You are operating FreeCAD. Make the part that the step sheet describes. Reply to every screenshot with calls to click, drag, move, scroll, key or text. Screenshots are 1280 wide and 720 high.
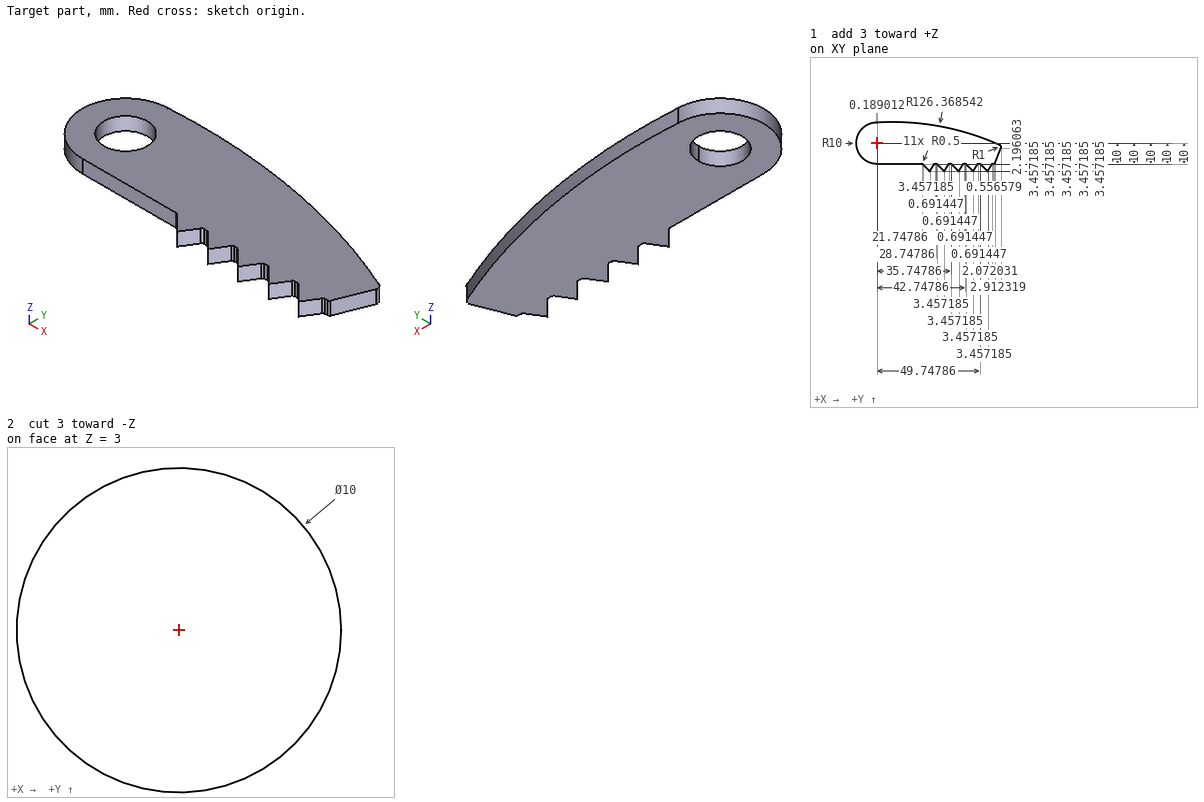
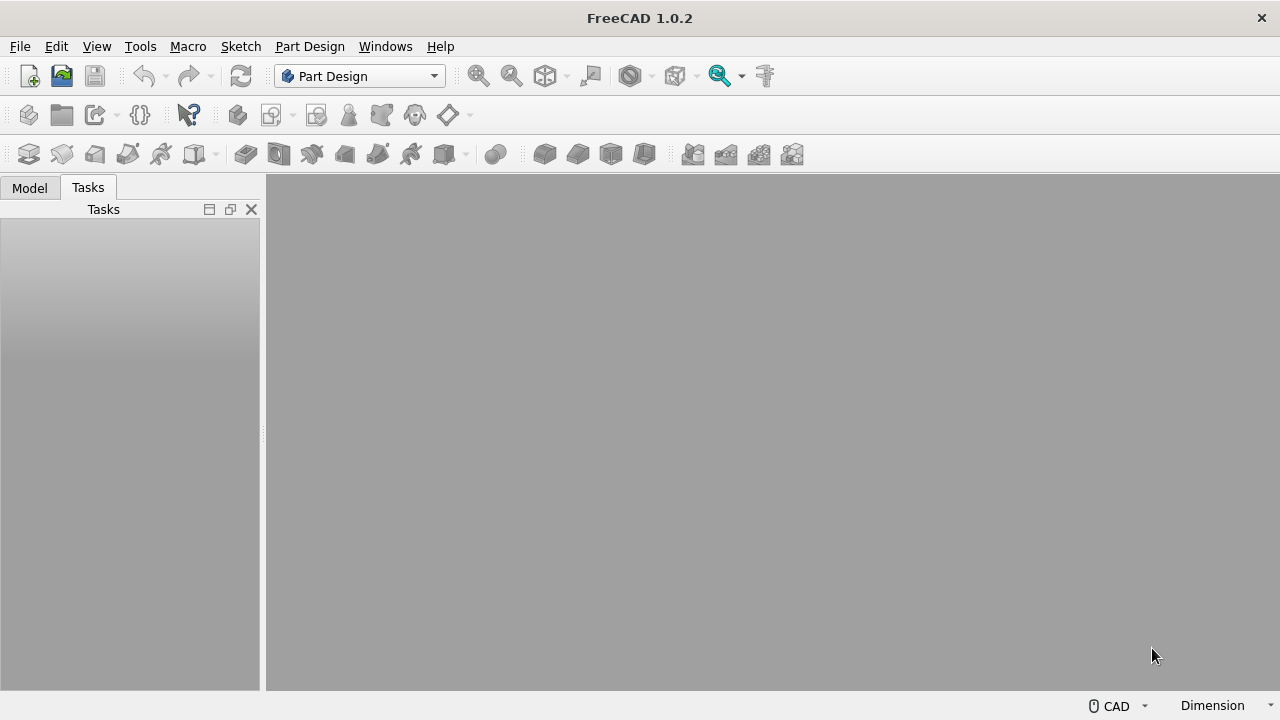
click(29, 76)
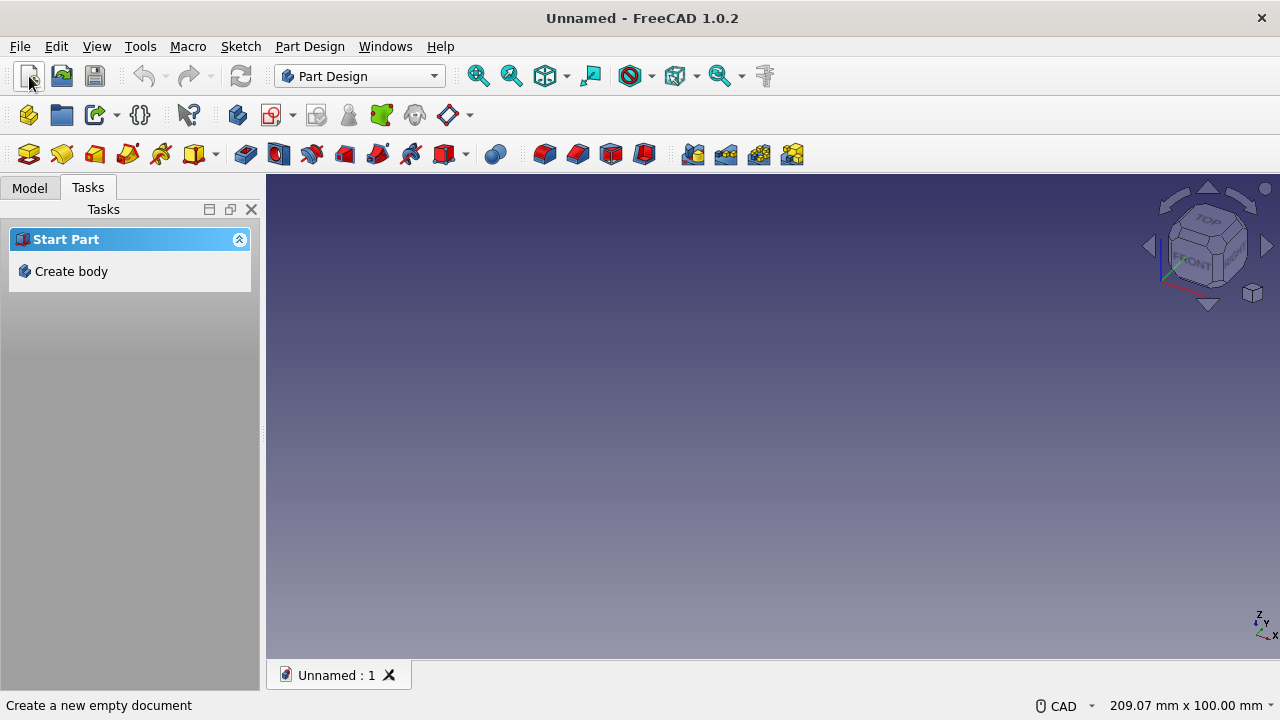
click(270, 116)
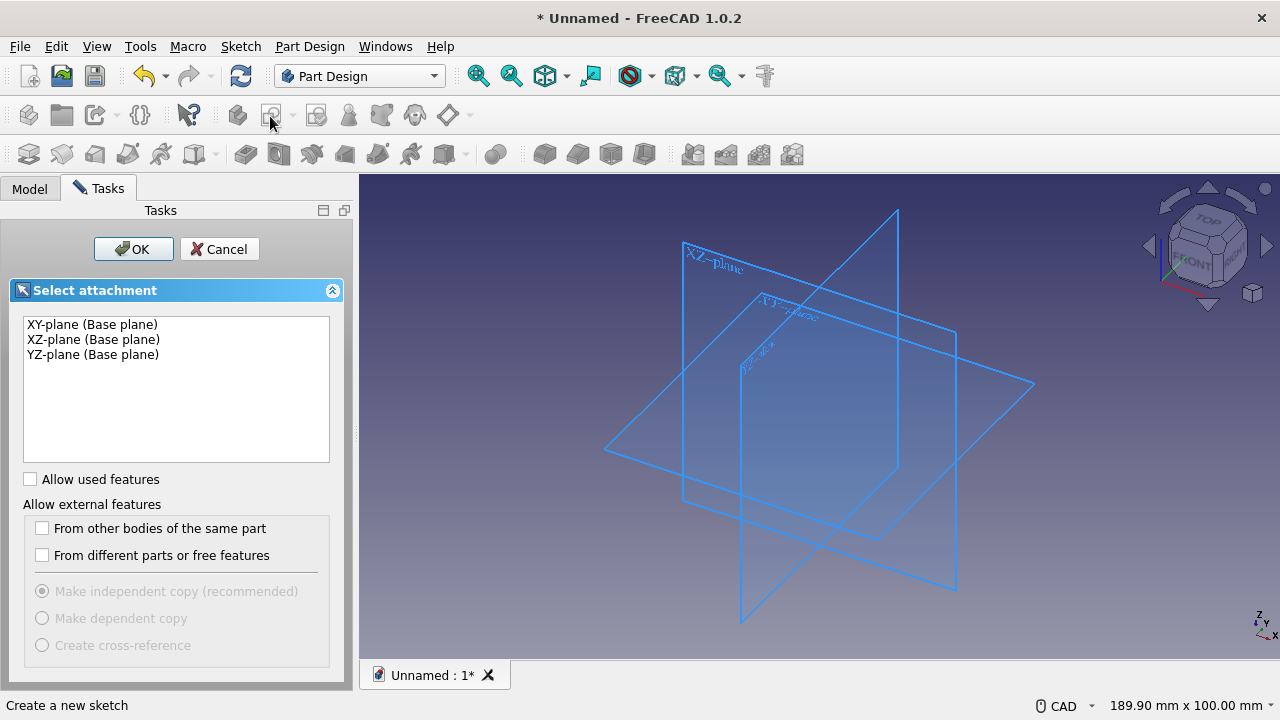
click(84, 324)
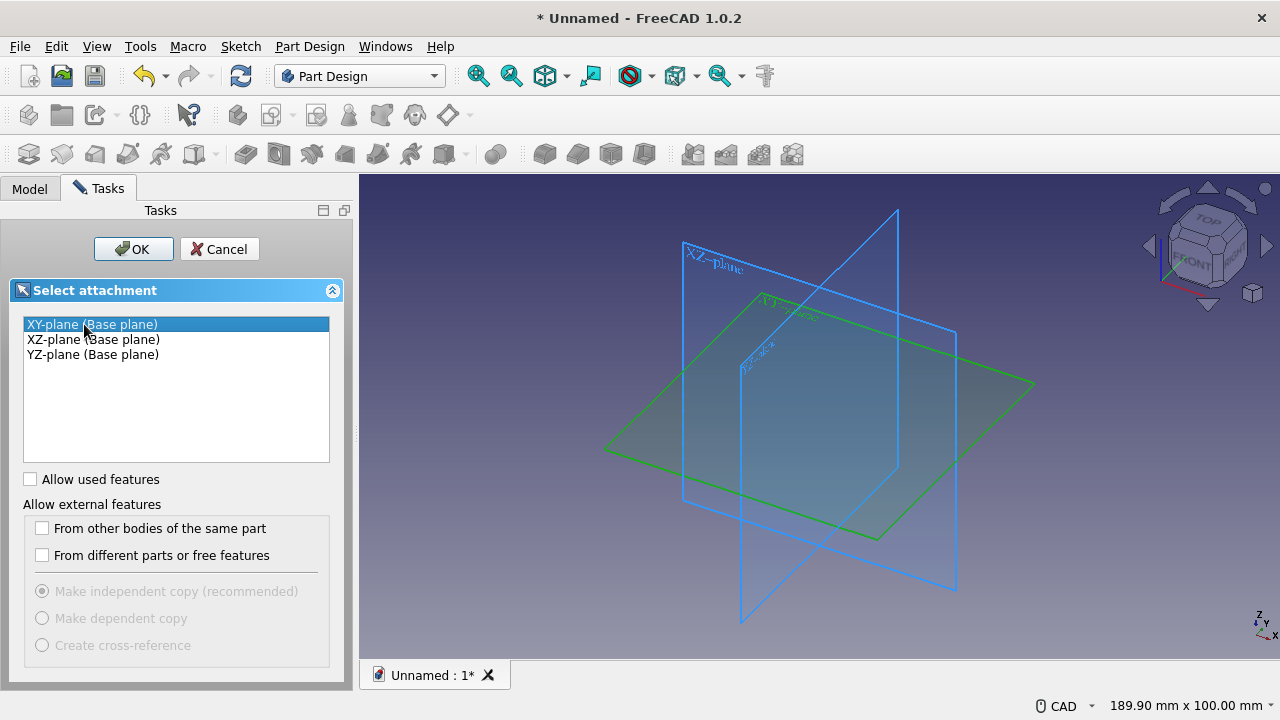
click(134, 249)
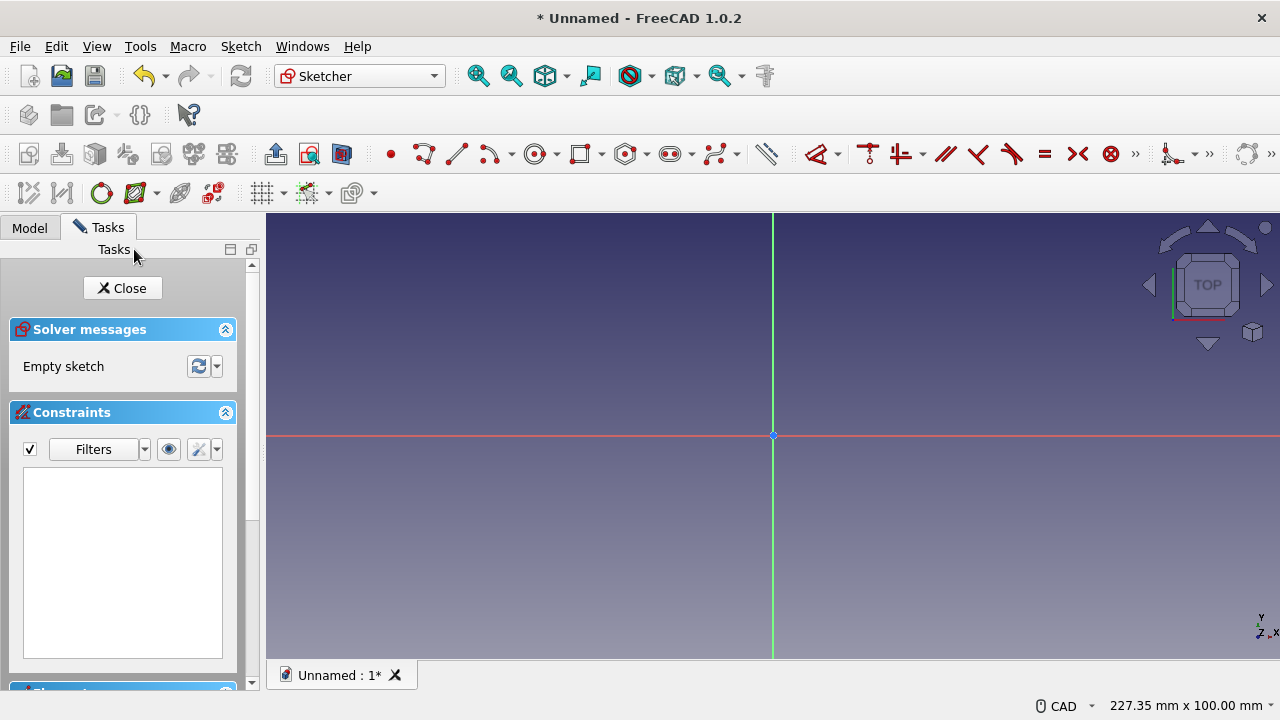
scroll(1103, 454, up, 3)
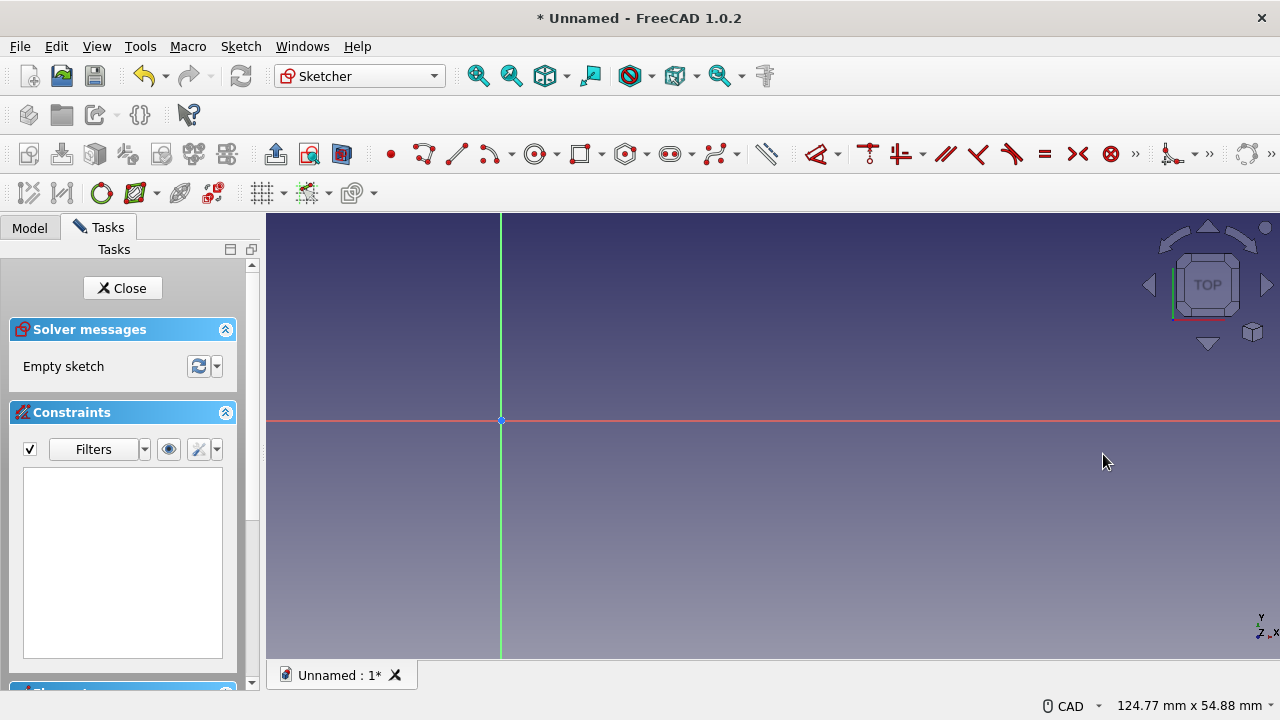
click(457, 154)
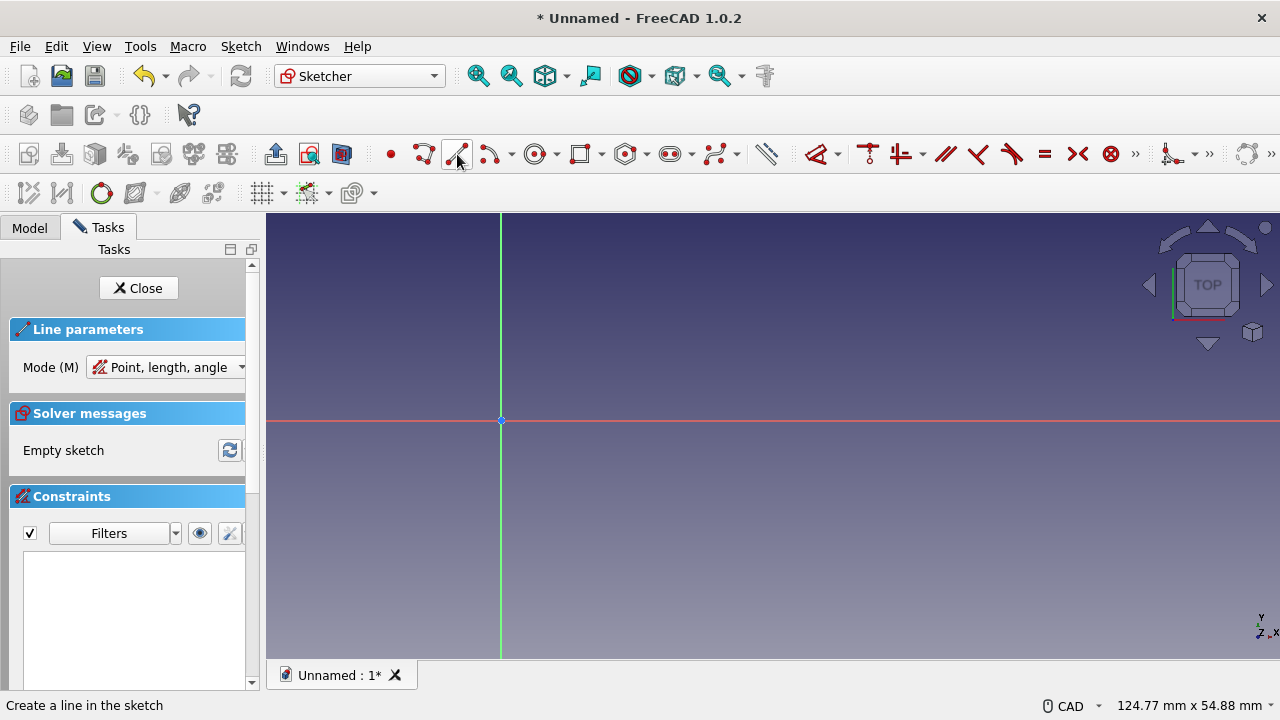
click(501, 502)
click(678, 502)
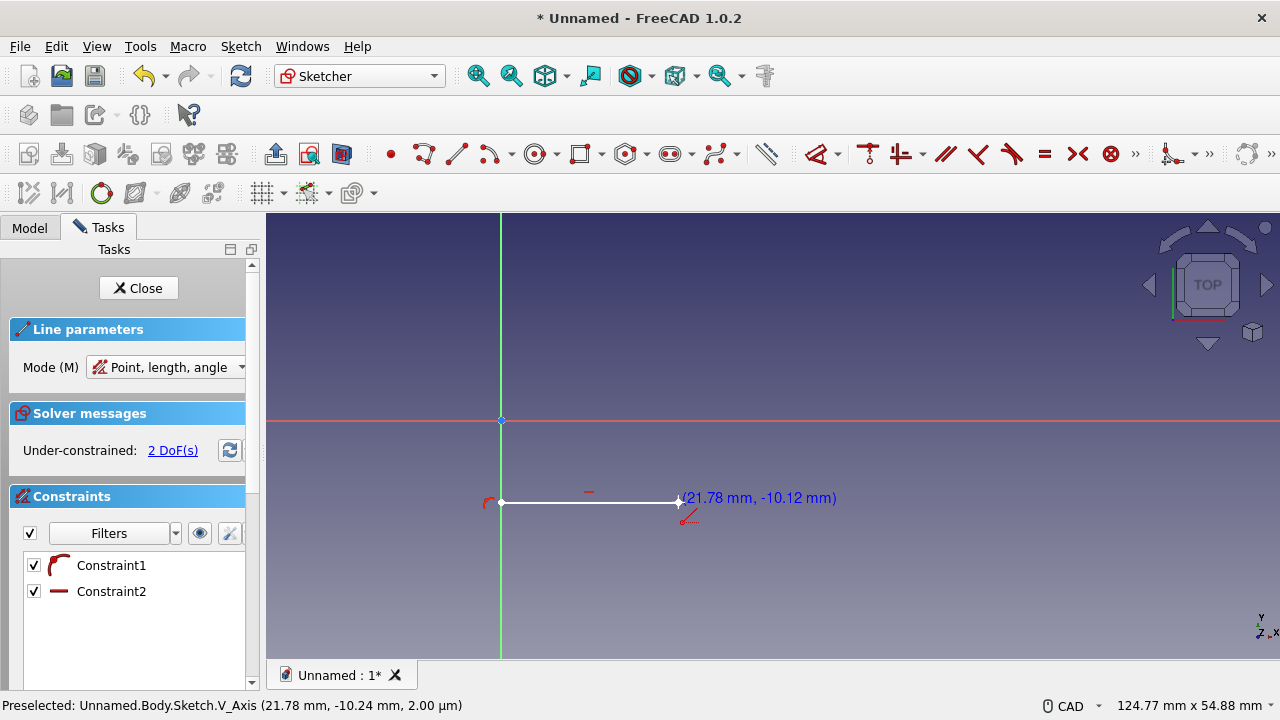
click(424, 154)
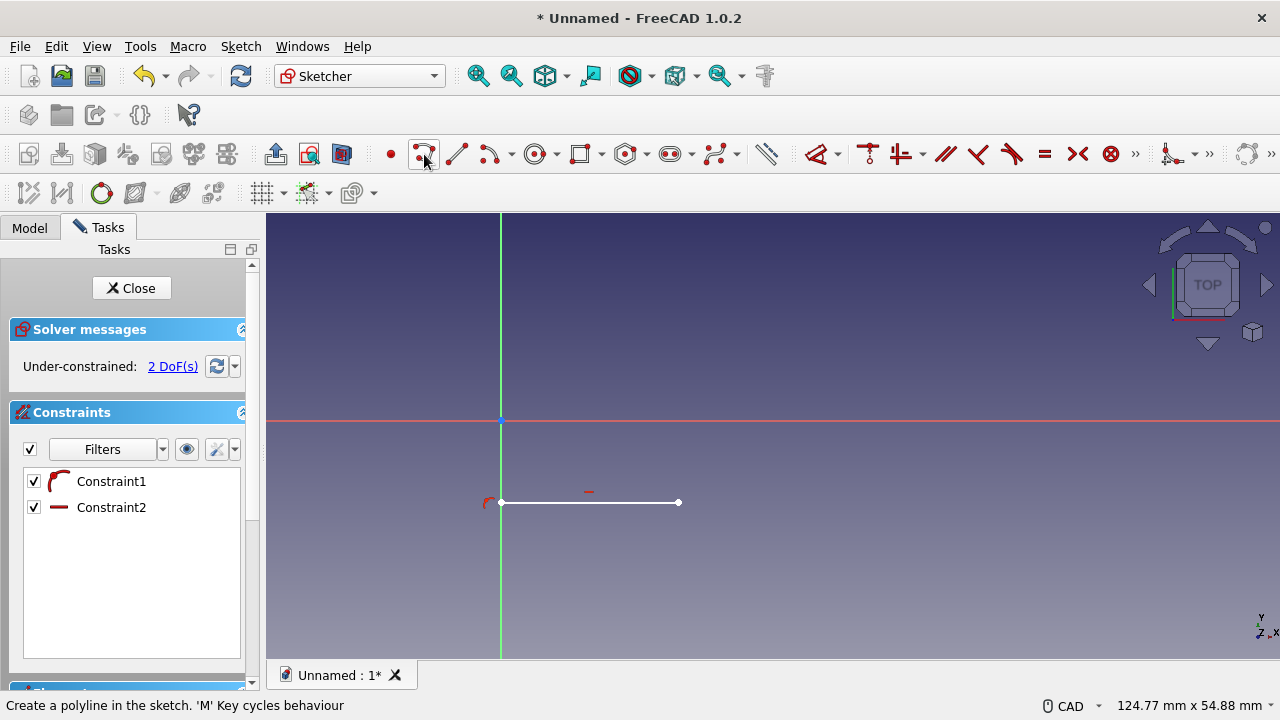
scroll(681, 503, up, 9)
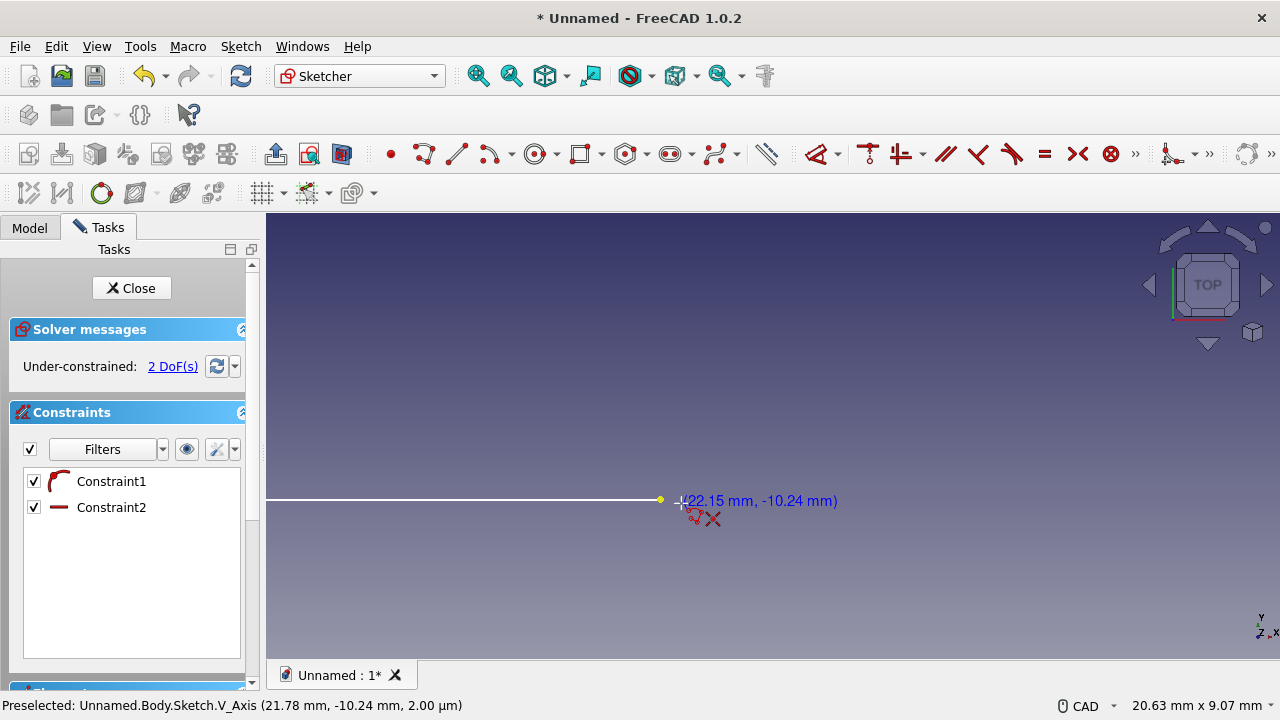
click(677, 501)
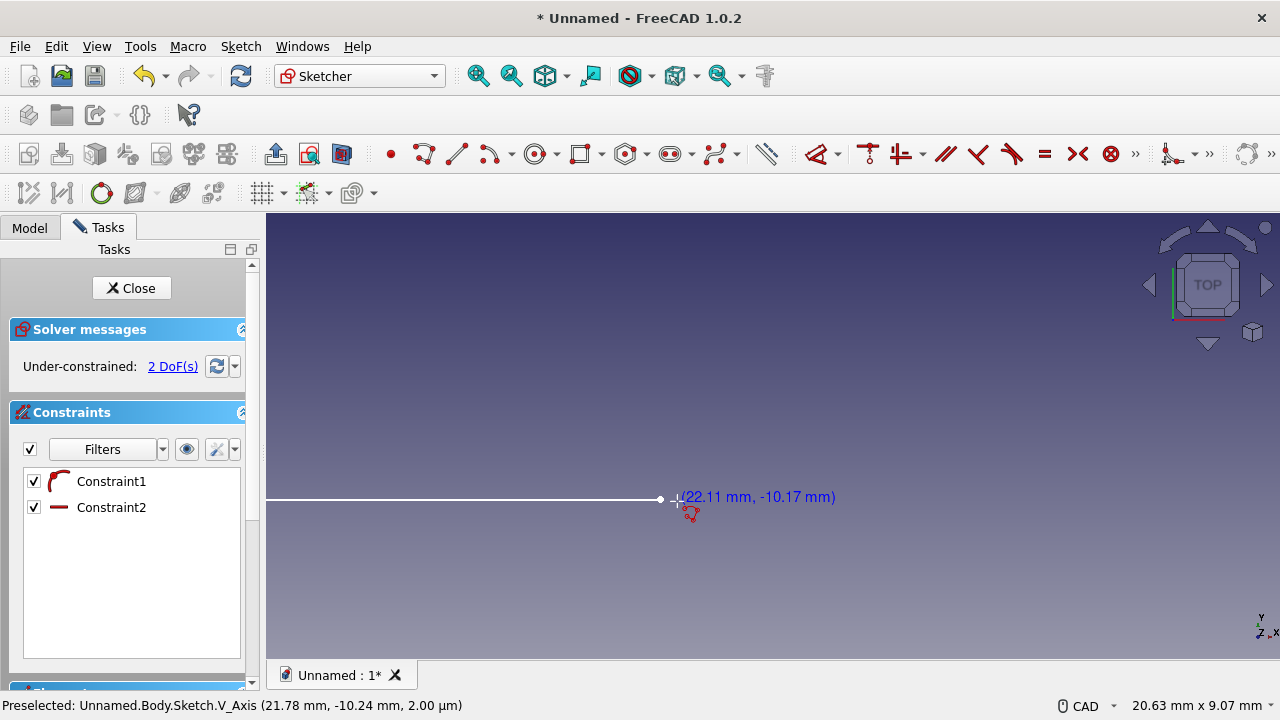
scroll(682, 504, down, 9)